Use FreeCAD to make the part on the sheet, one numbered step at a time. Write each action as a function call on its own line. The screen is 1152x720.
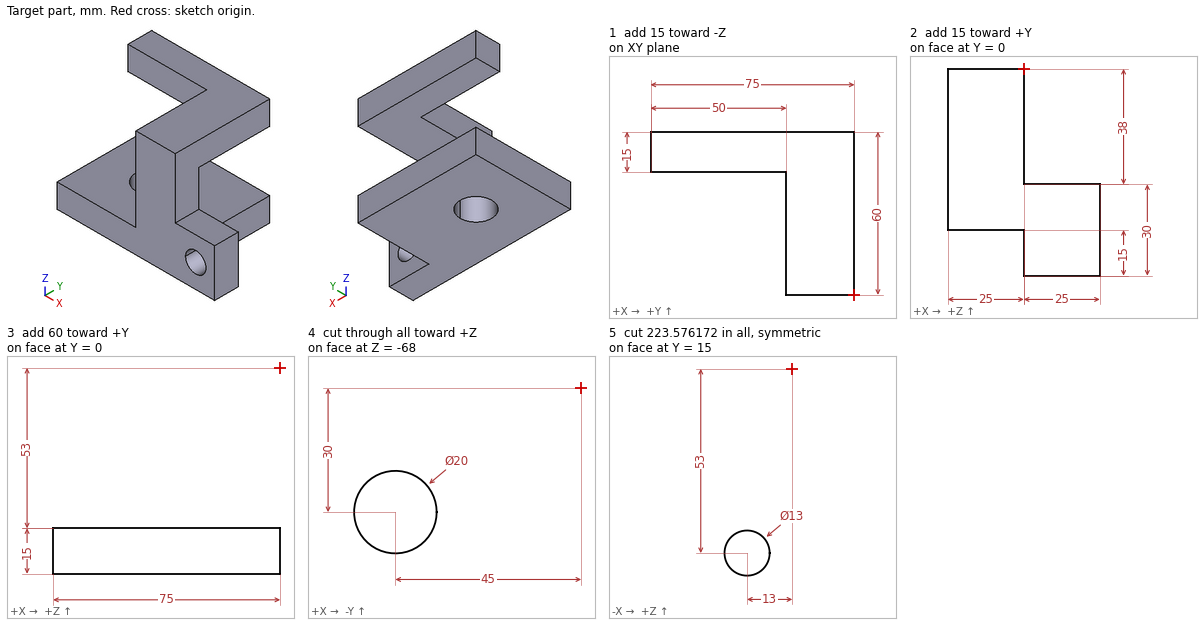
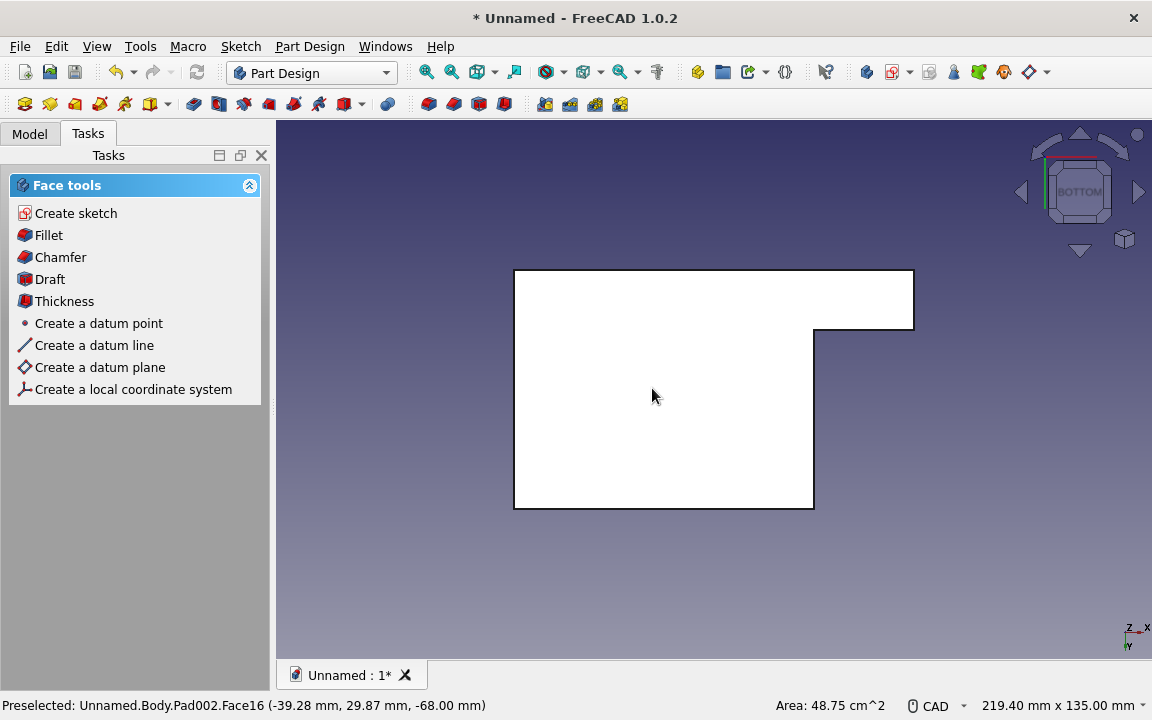
click(892, 72)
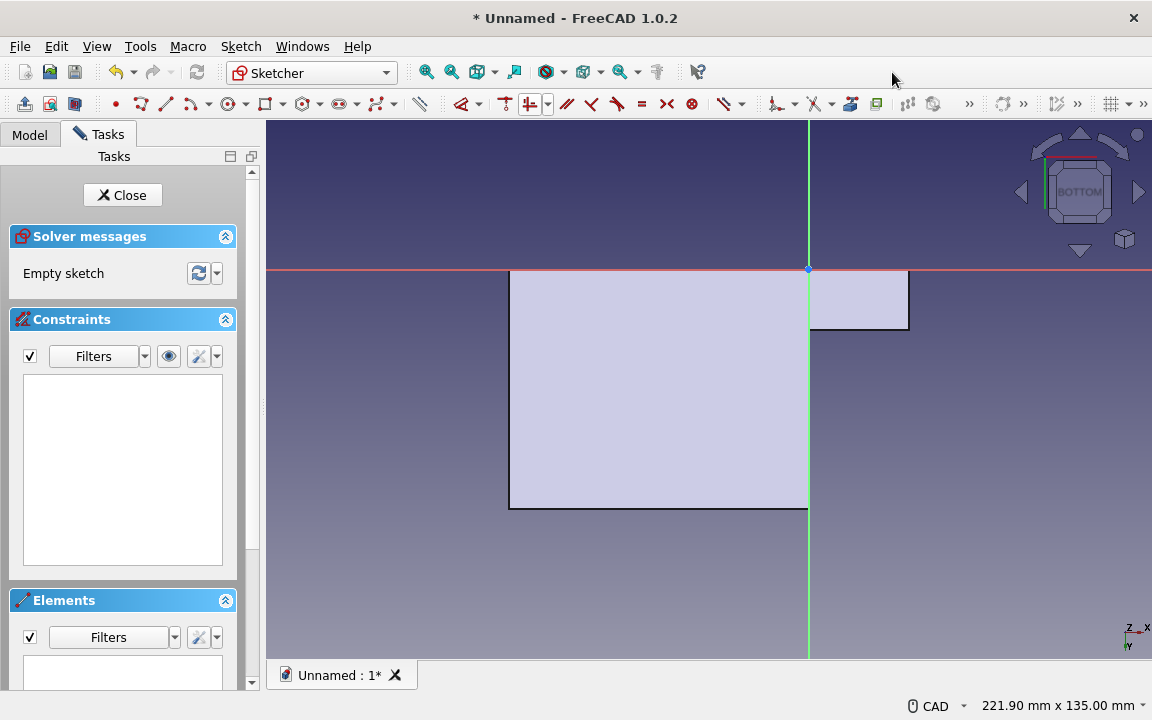
scroll(625, 389, up, 7)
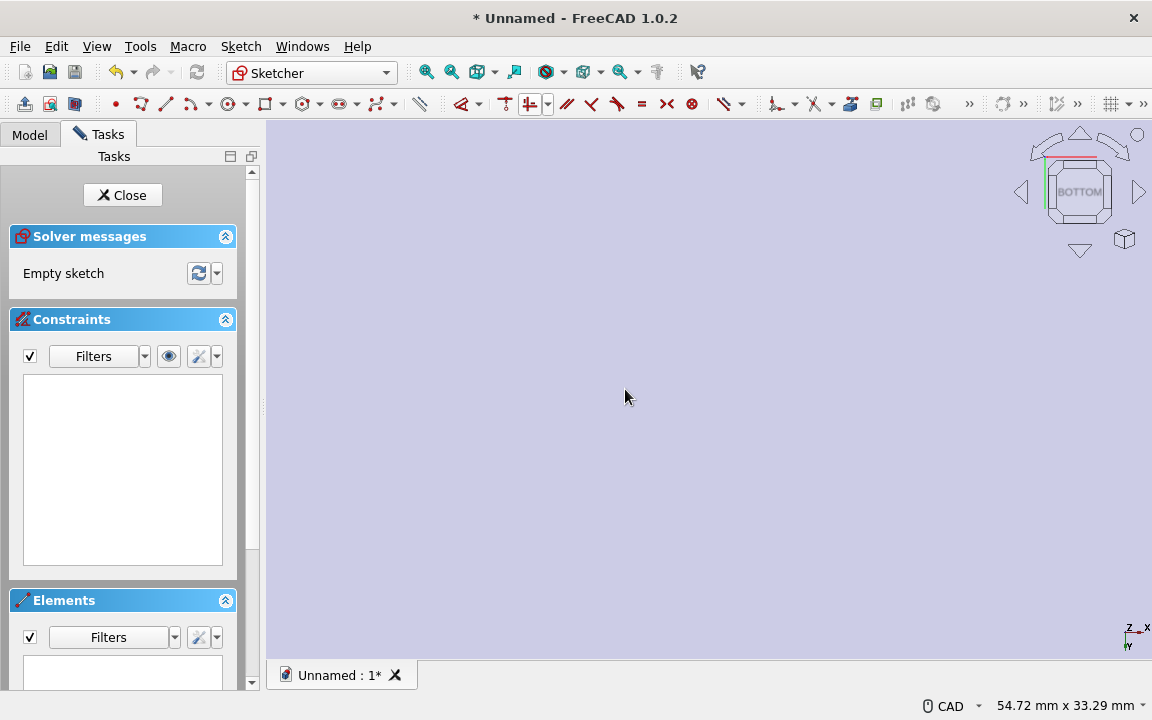
key(g)
key(c)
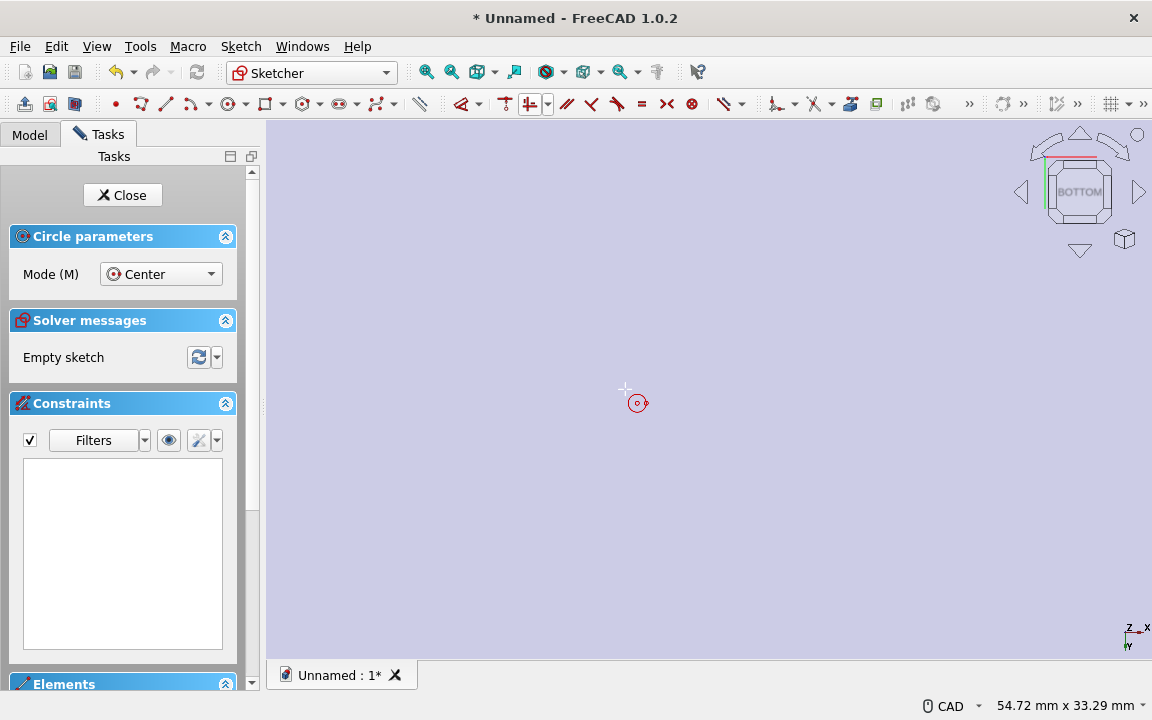
click(641, 389)
click(755, 275)
key(Escape)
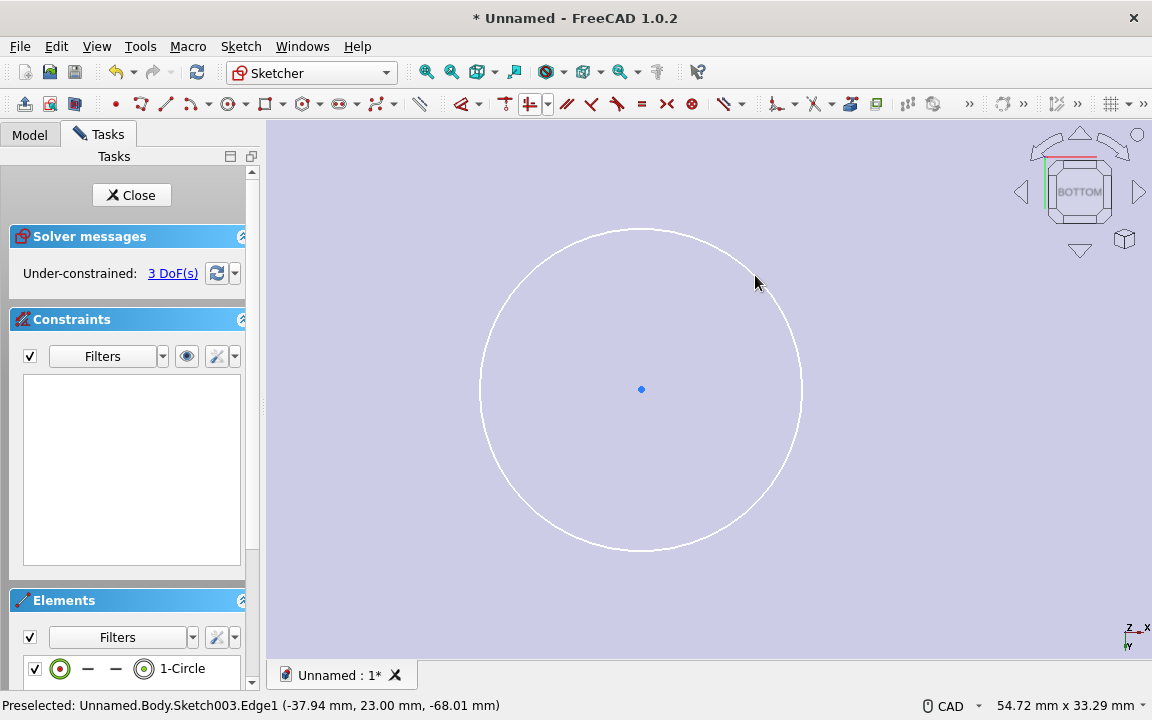
click(460, 104)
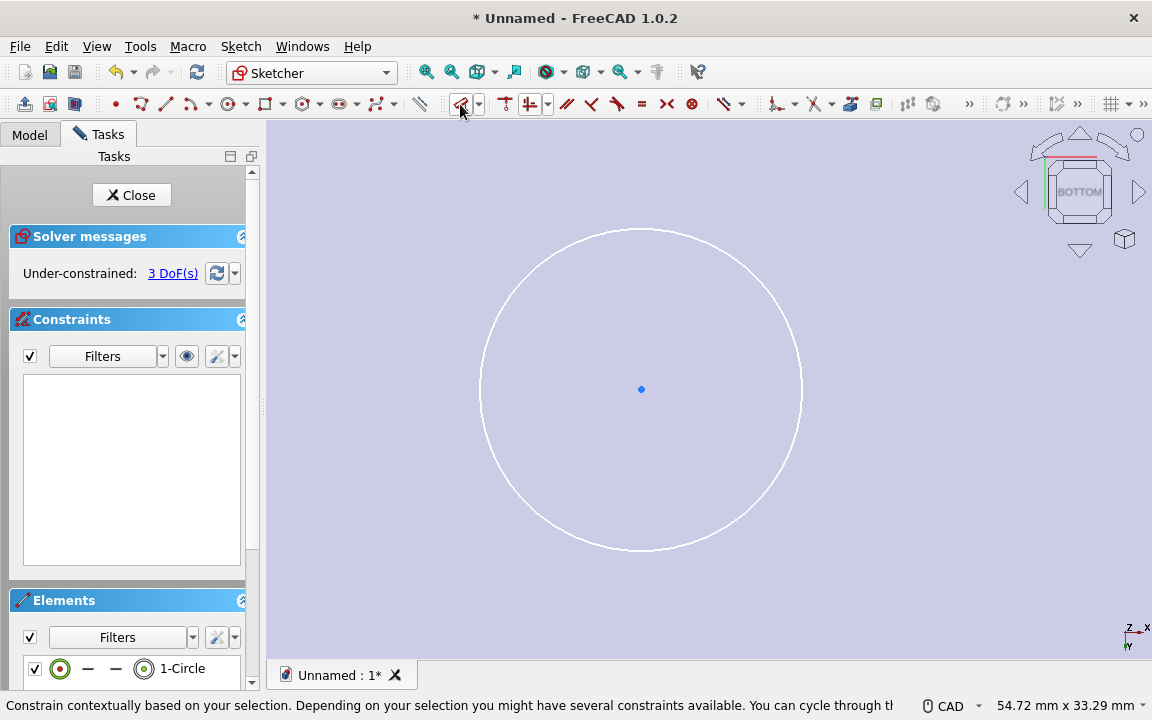
click(755, 276)
click(778, 253)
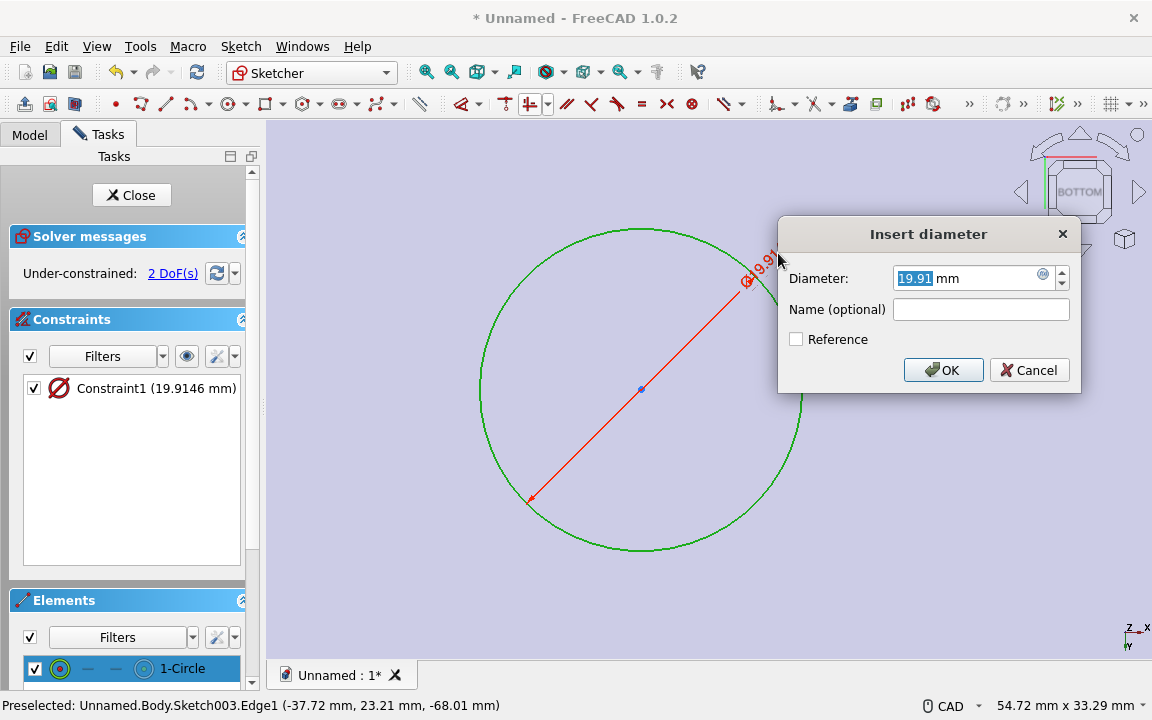
text(20)
key(Return)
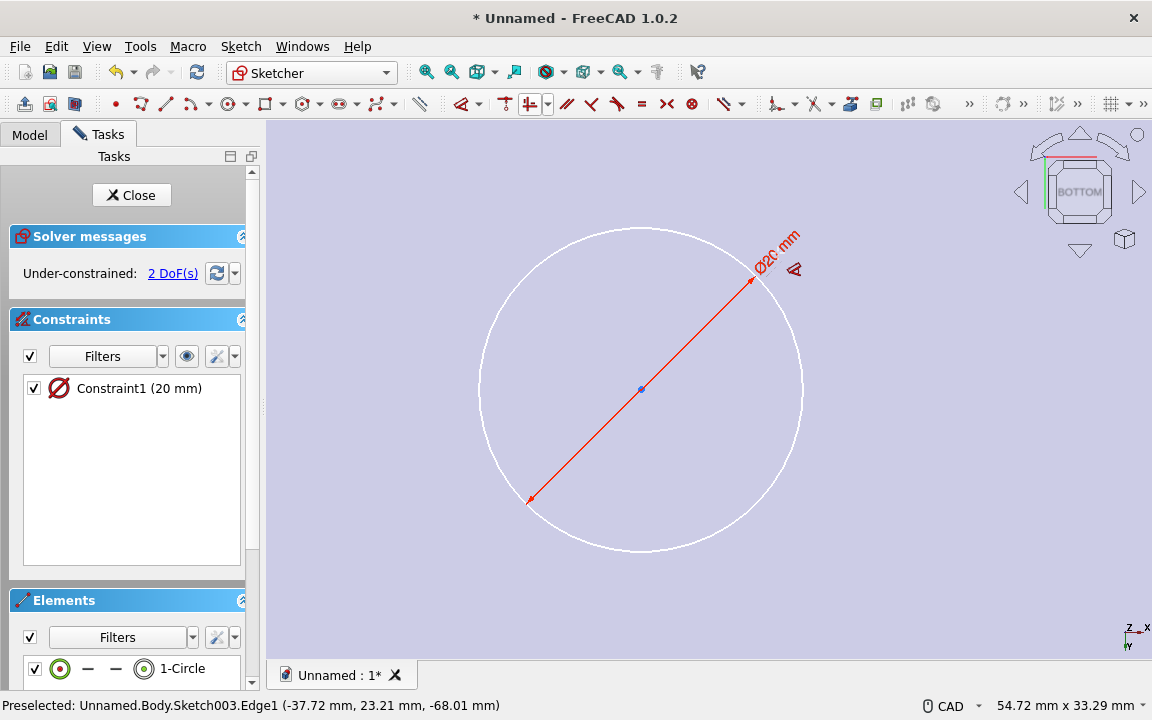
click(641, 390)
click(814, 424)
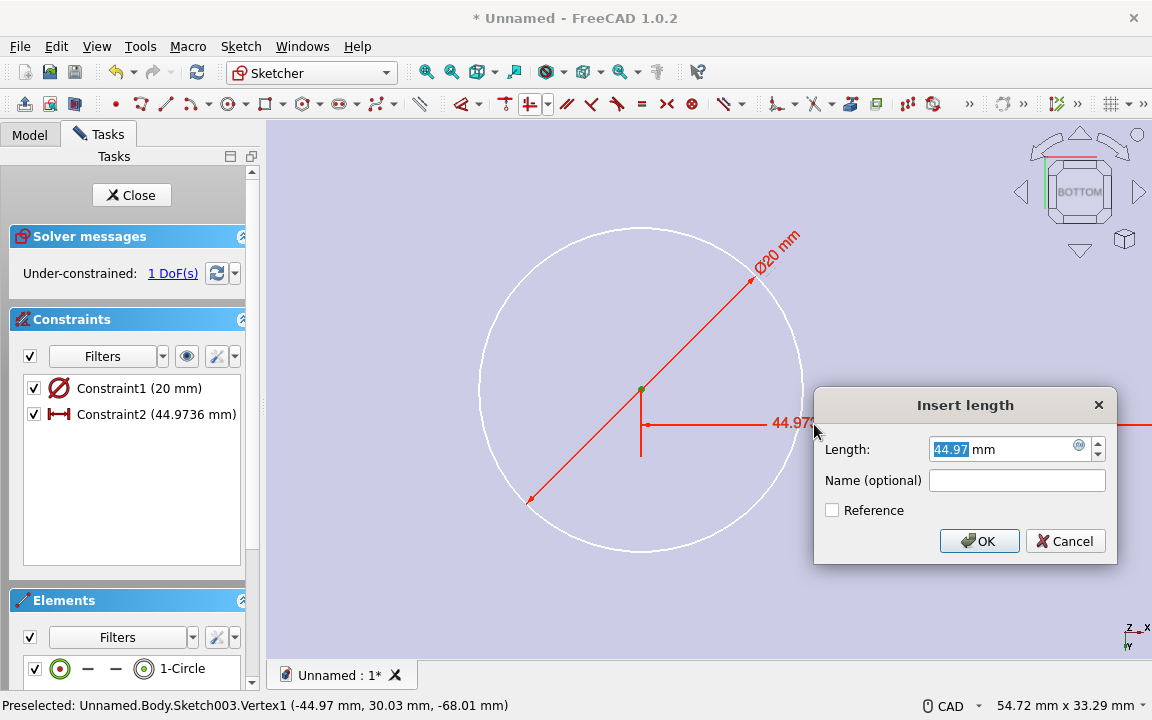
text(45)
key(Return)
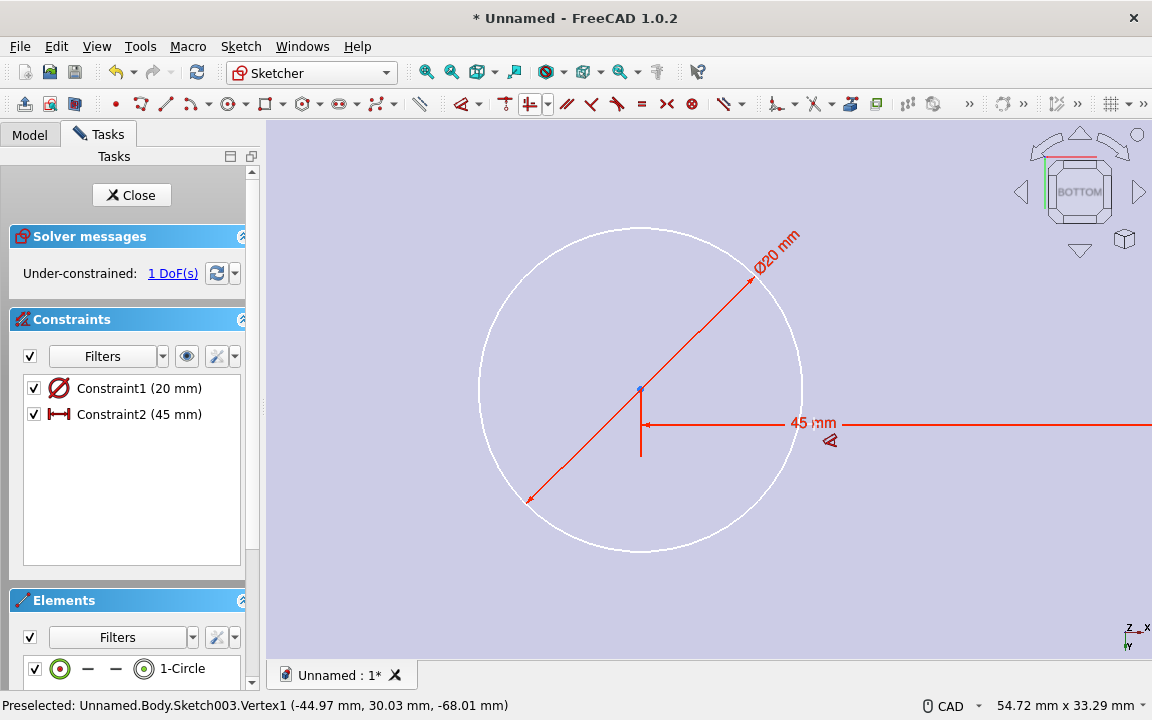
click(641, 390)
click(607, 269)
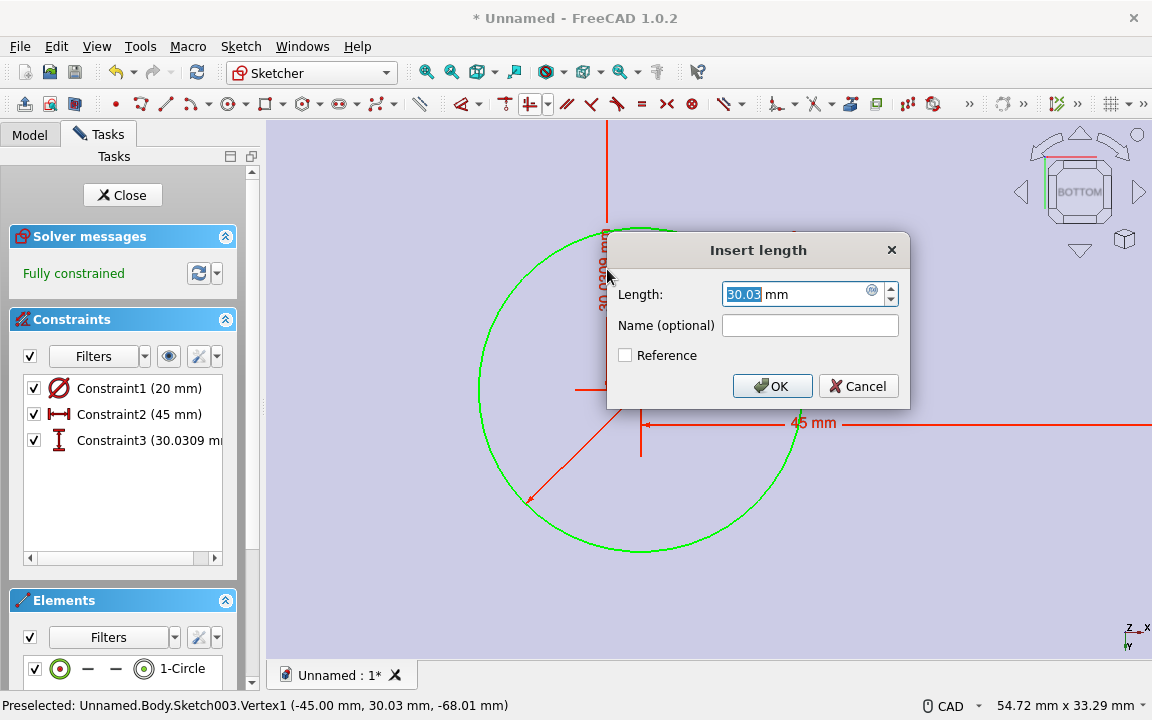
text(30)
key(Return)
key(Escape)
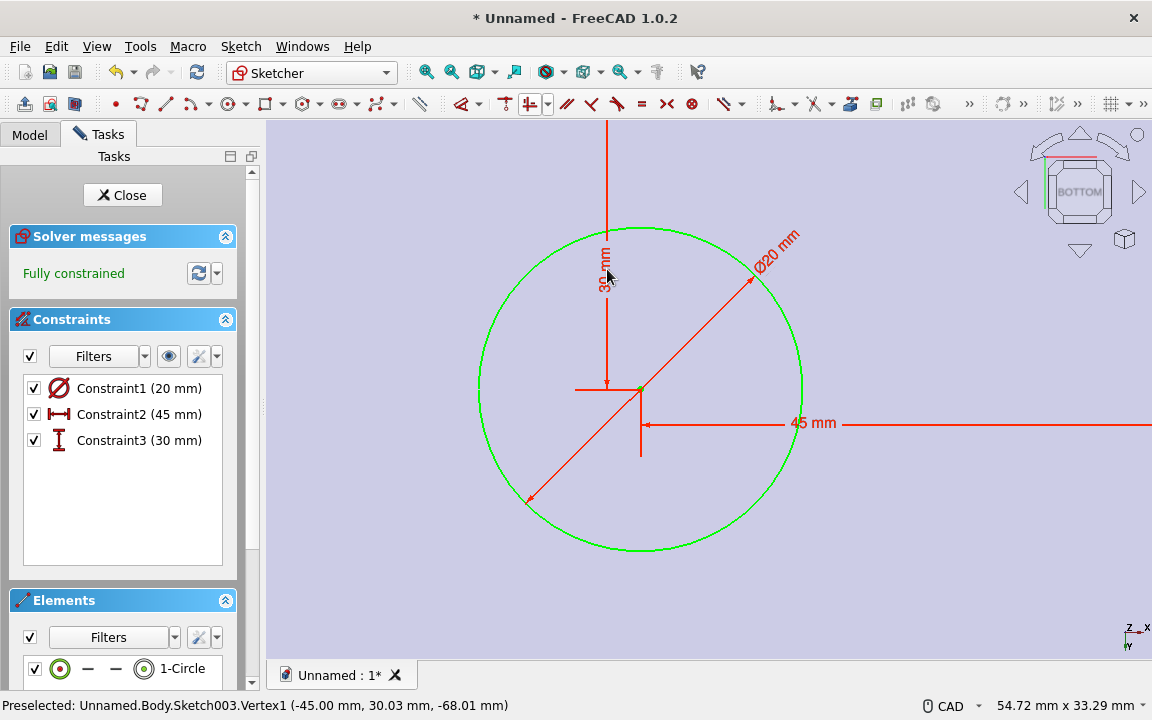
click(123, 195)